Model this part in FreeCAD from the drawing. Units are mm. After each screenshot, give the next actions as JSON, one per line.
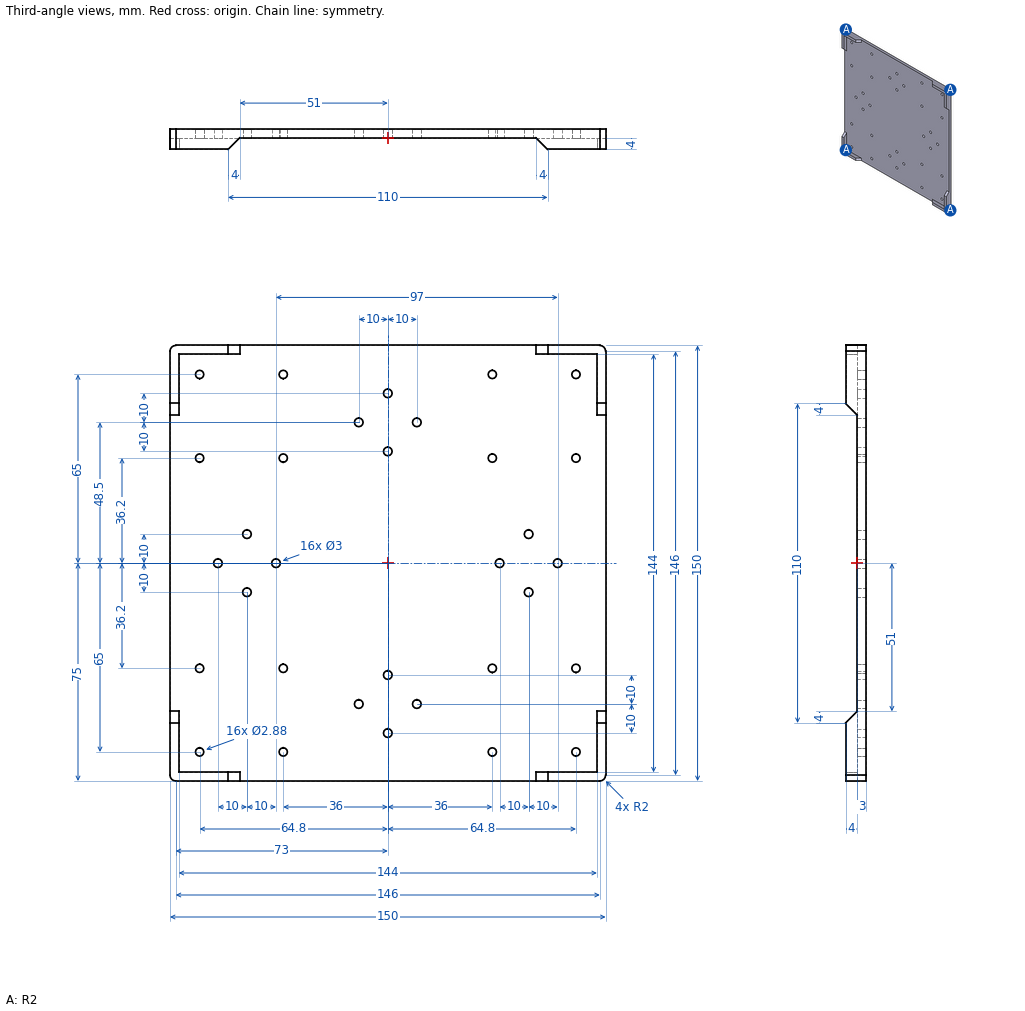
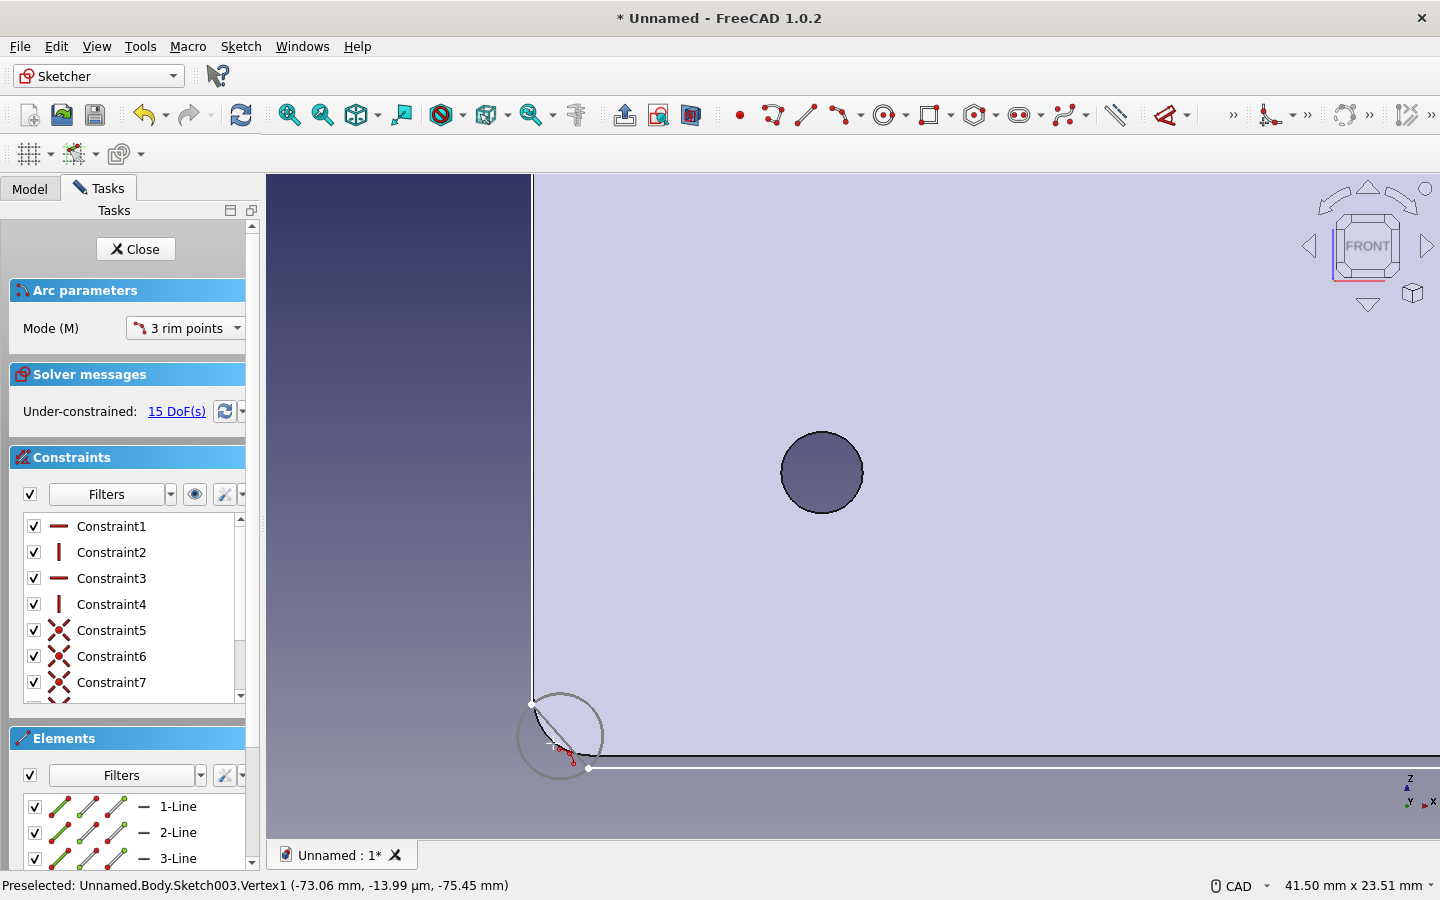
{"action": "left_click", "coordinate": [550, 739]}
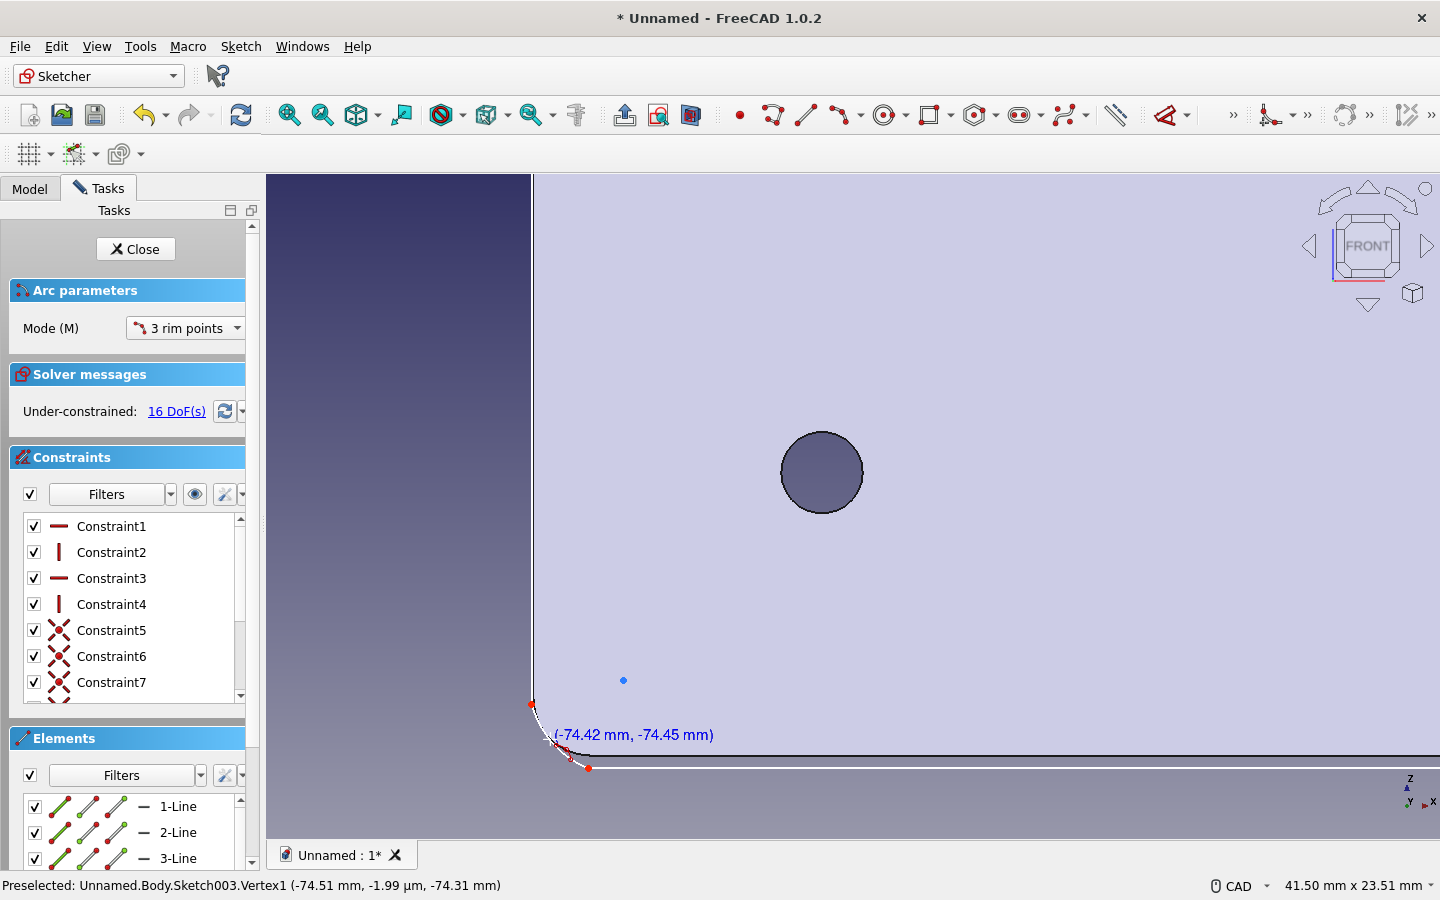
{"action": "key", "text": "g v"}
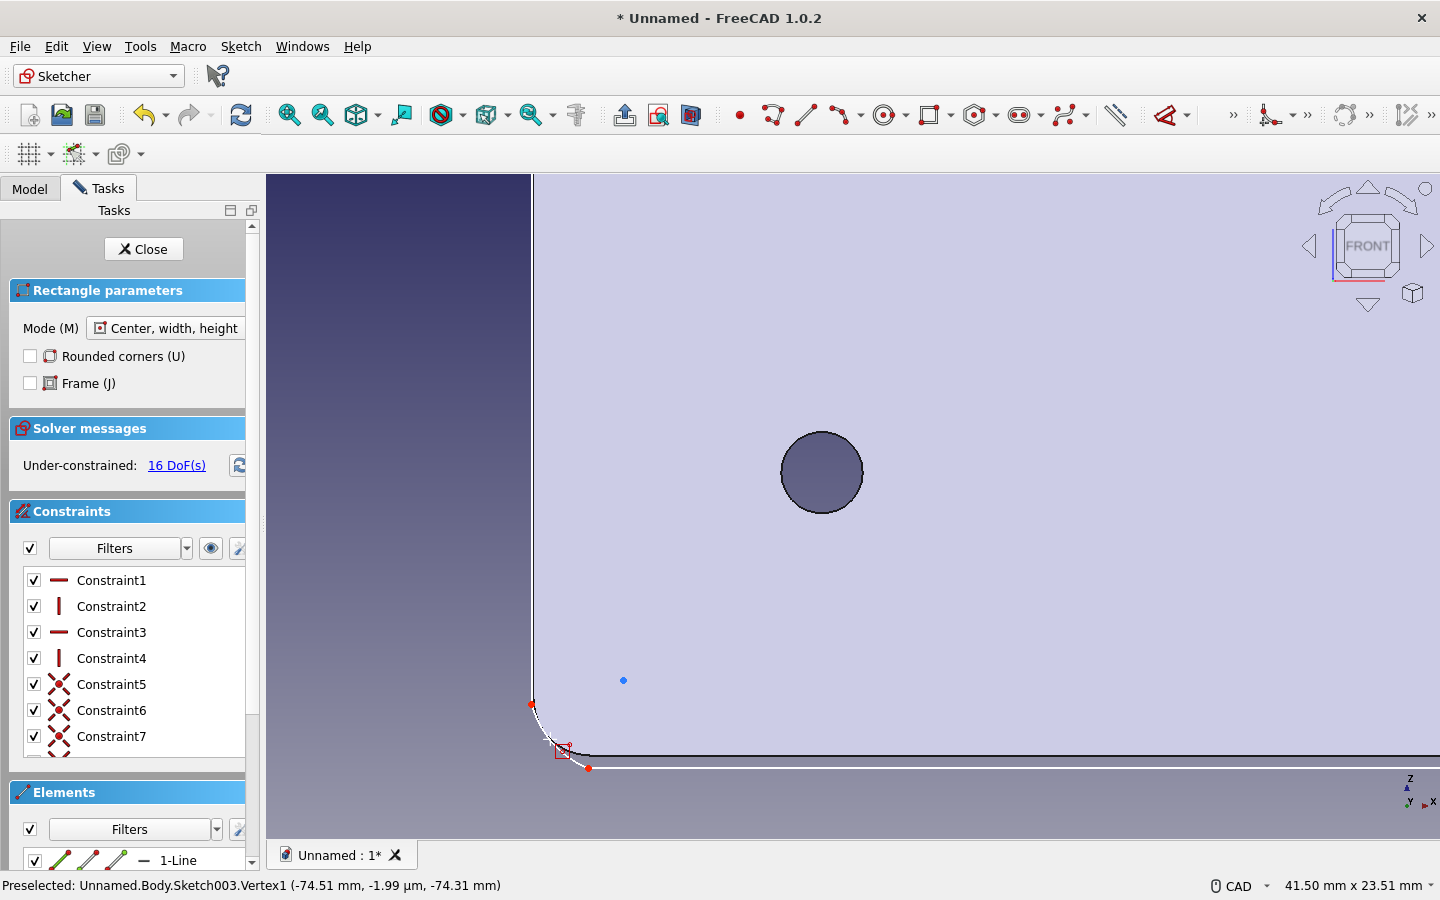
{"action": "scroll", "coordinate": [551, 740], "scroll_direction": "down", "scroll_amount": 11}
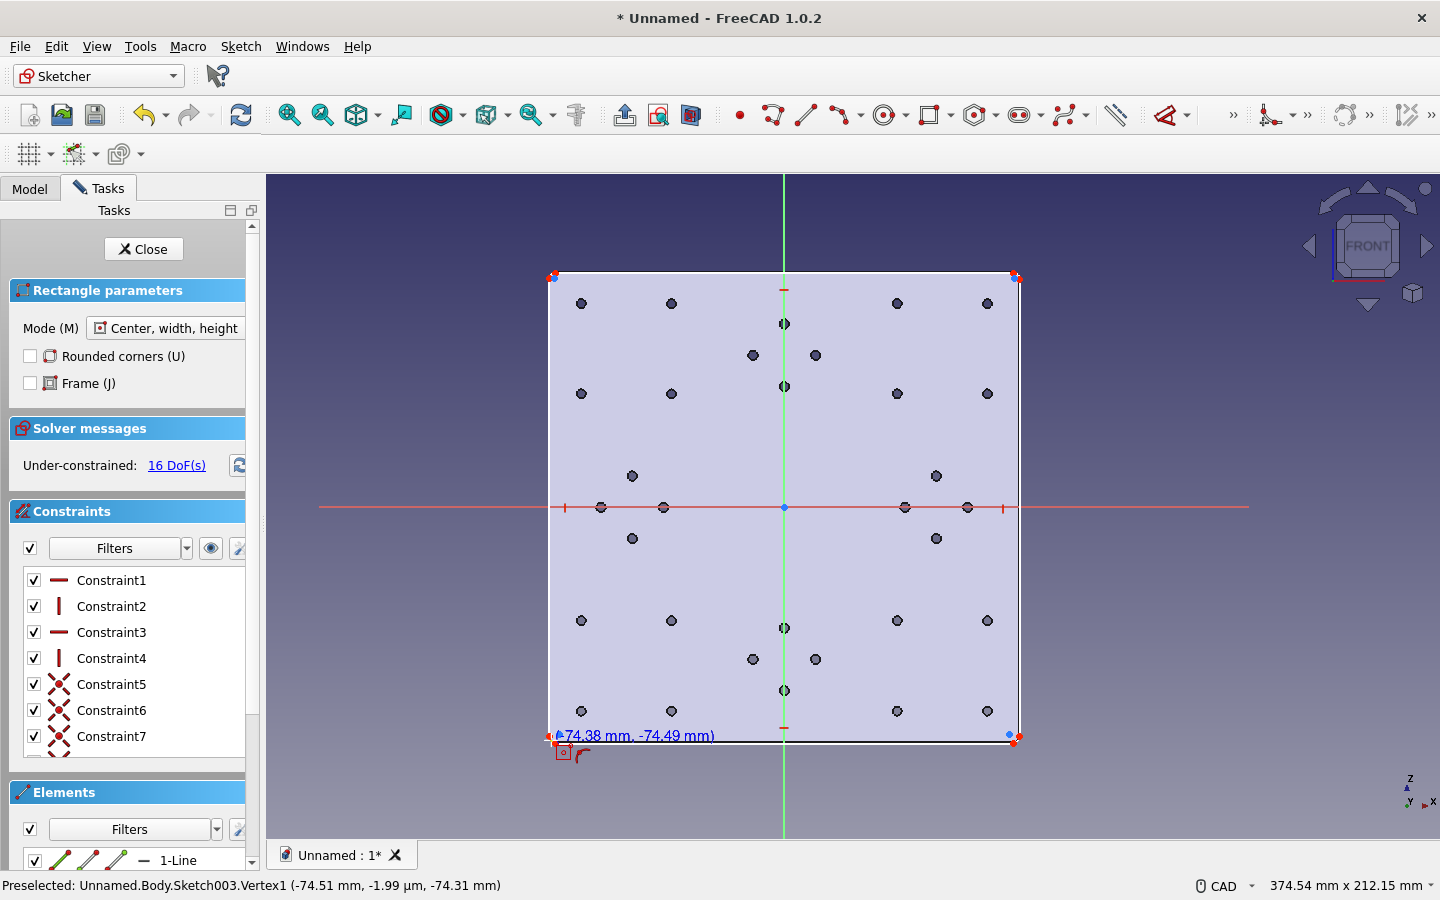
{"action": "left_click", "coordinate": [784, 507]}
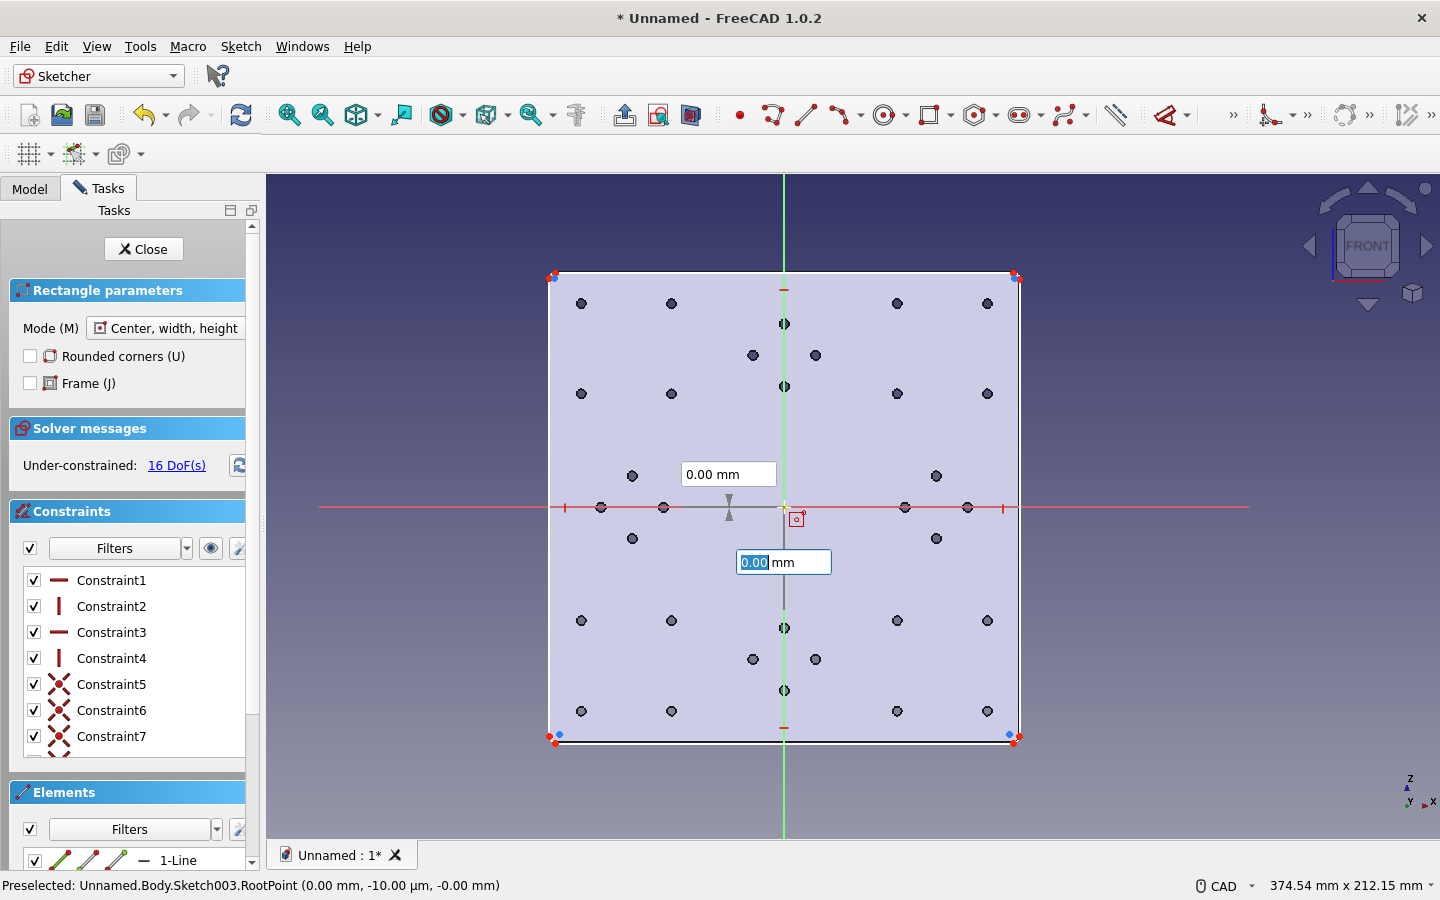
{"action": "scroll", "coordinate": [1010, 282], "scroll_direction": "up", "scroll_amount": 7}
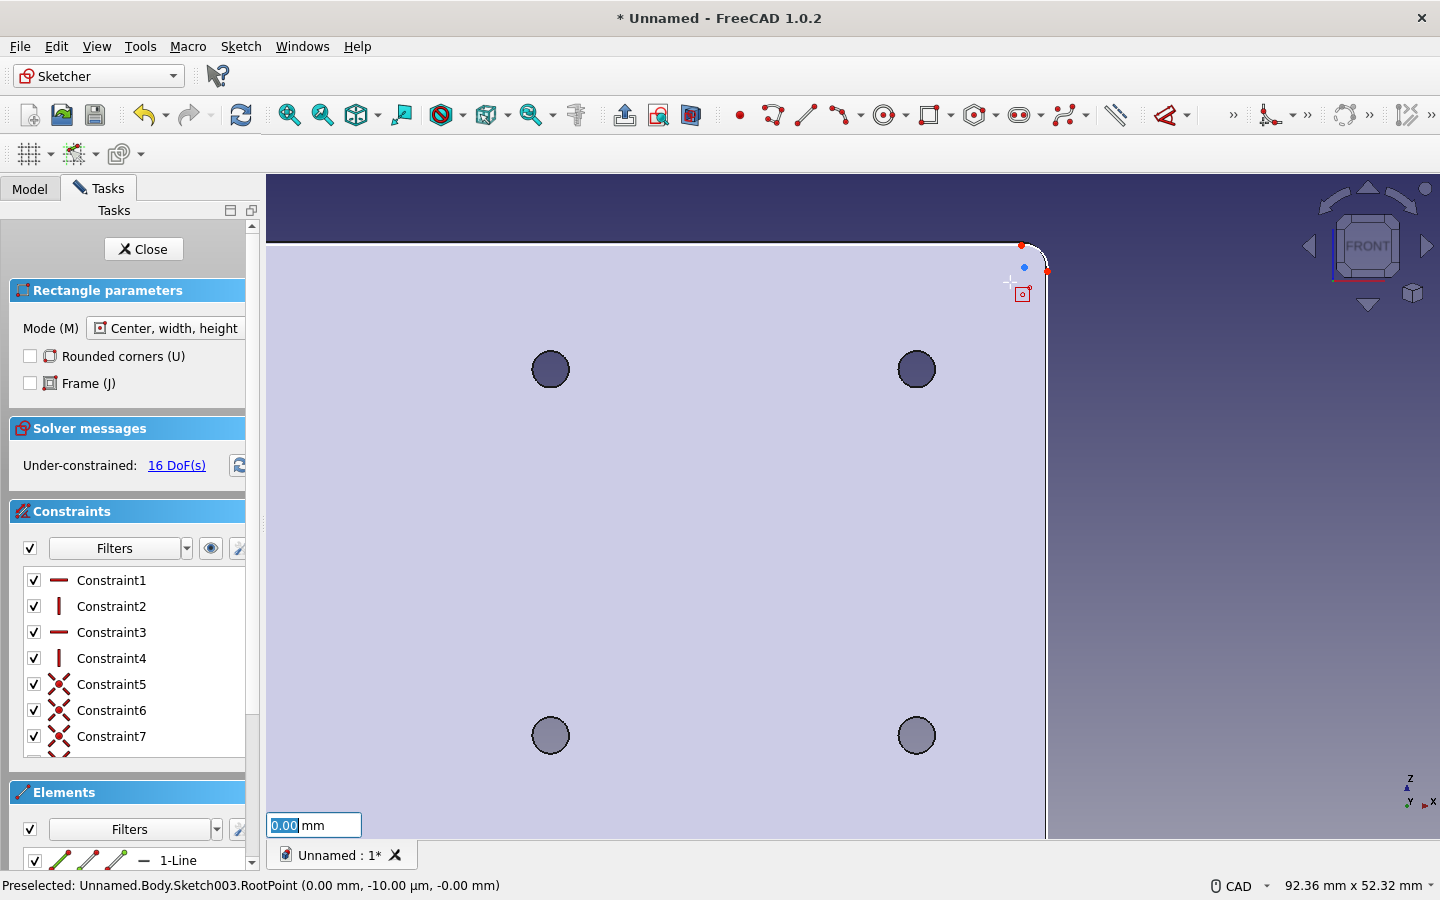
{"action": "left_click", "coordinate": [1008, 280]}
{"action": "key", "text": "Escape"}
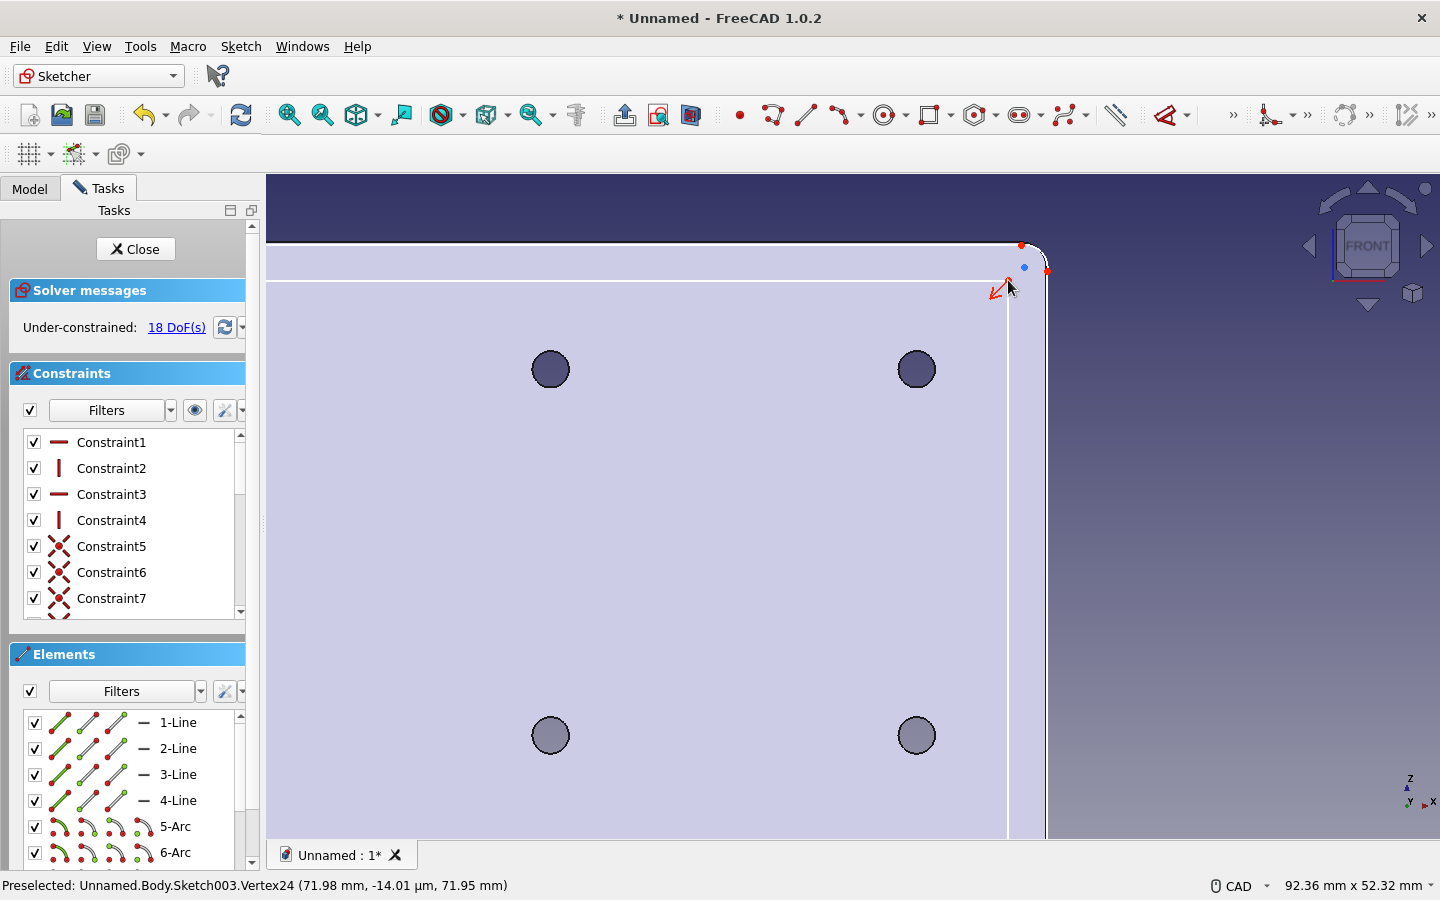
{"action": "scroll", "coordinate": [1011, 281], "scroll_direction": "down", "scroll_amount": 7}